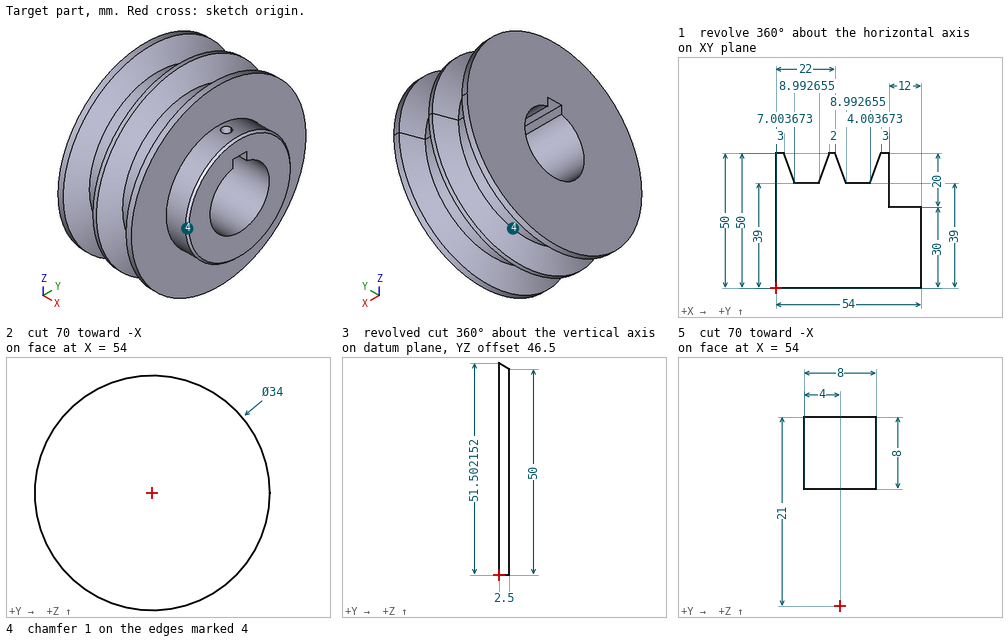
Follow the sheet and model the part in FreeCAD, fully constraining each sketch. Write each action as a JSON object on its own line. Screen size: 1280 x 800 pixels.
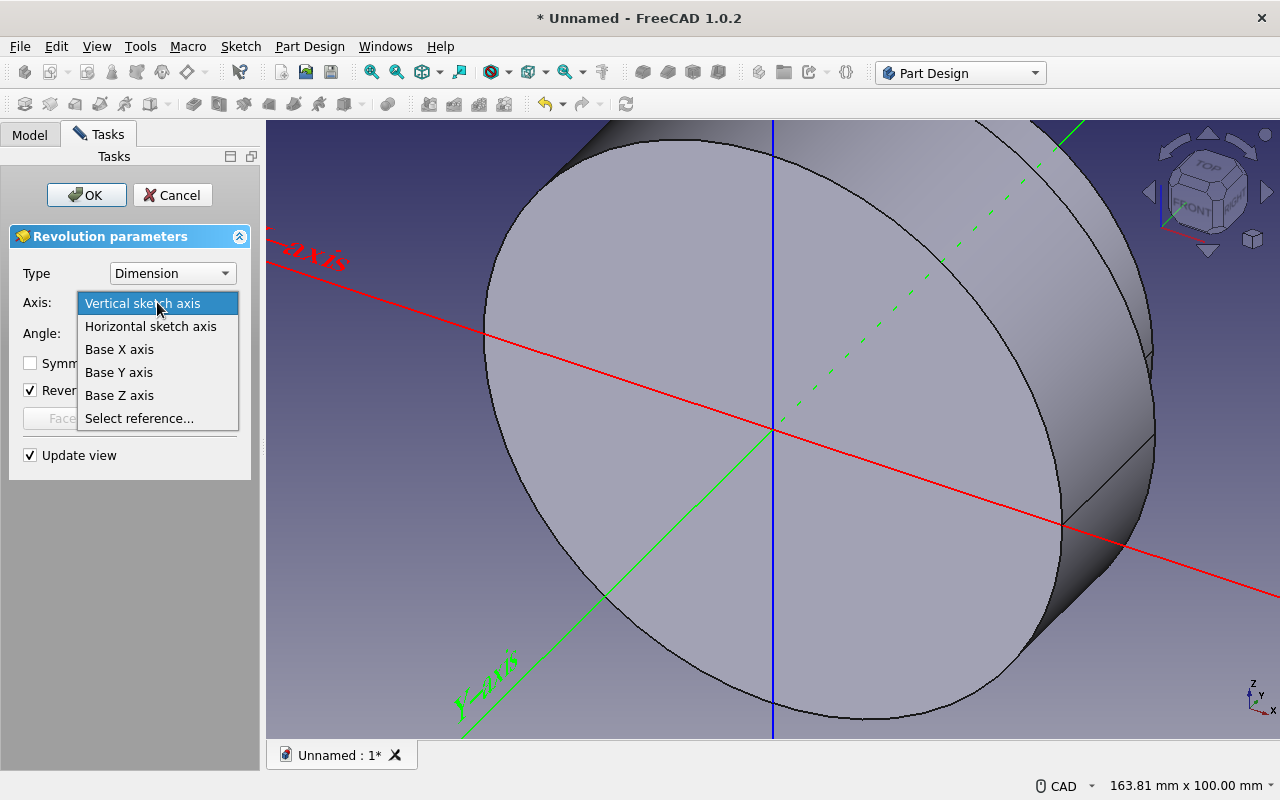
{"action": "left_click", "coordinate": [156, 326]}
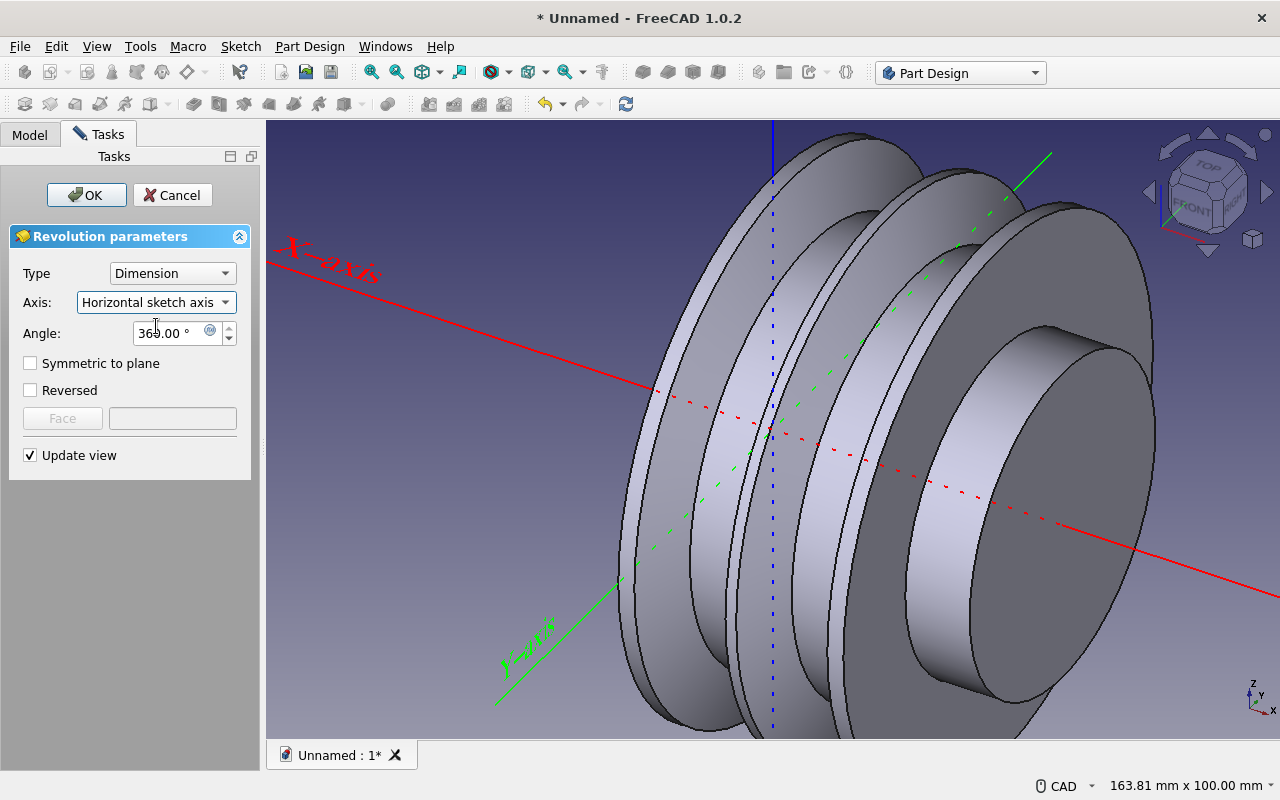
{"action": "left_click", "coordinate": [87, 195]}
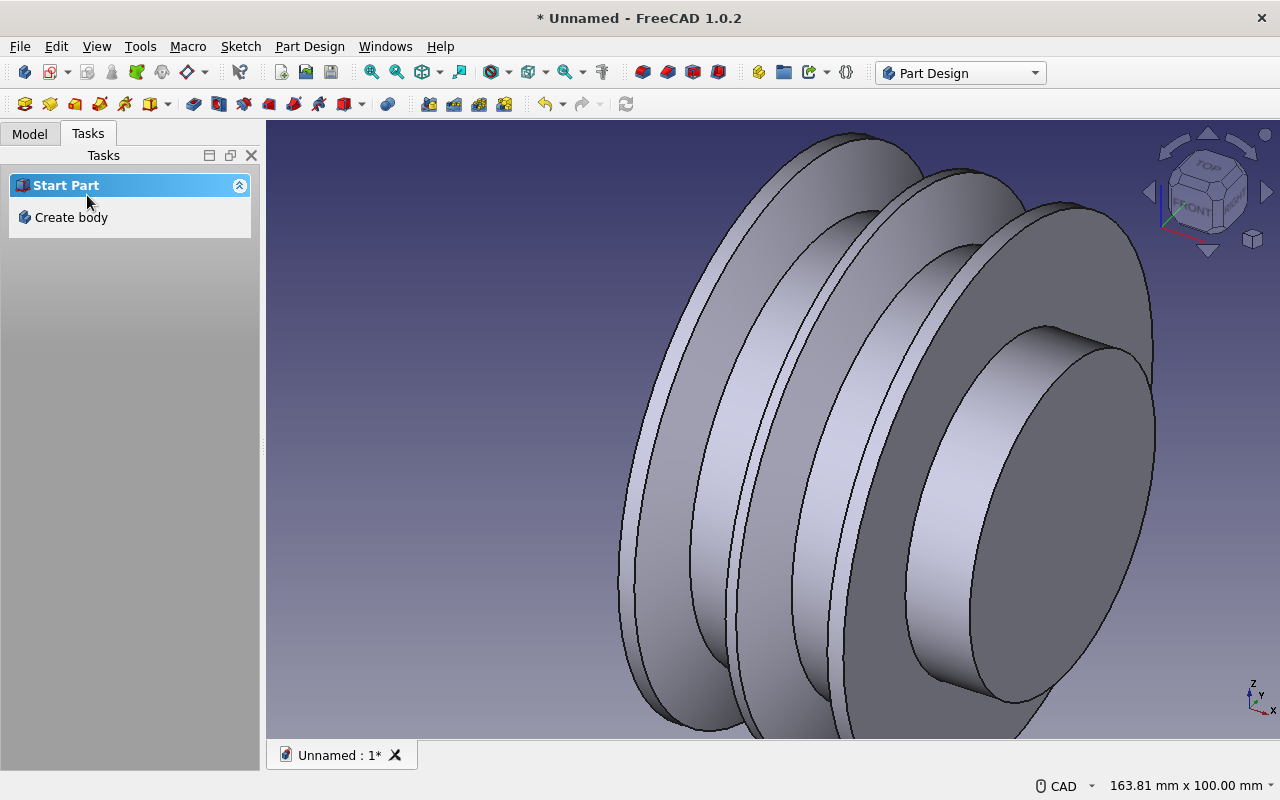
{"action": "key", "text": "v f"}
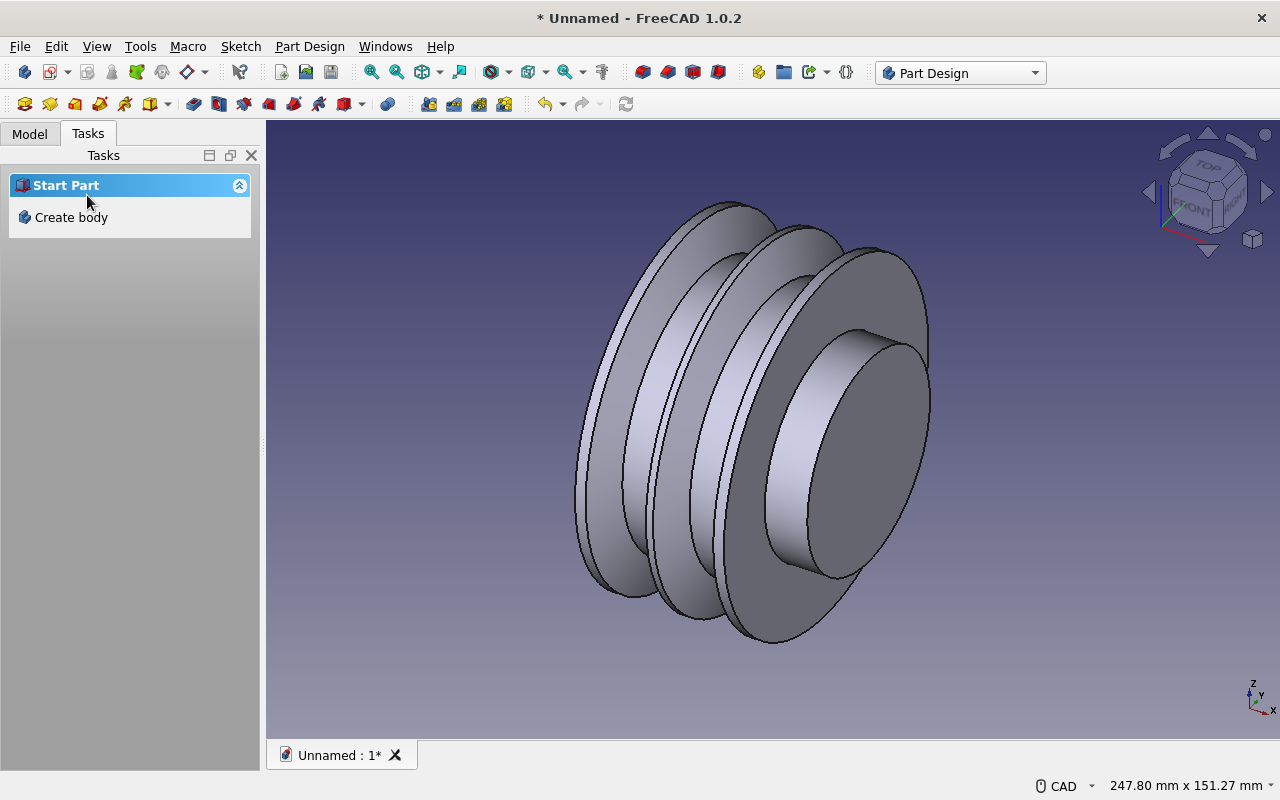
{"action": "left_click", "coordinate": [869, 460]}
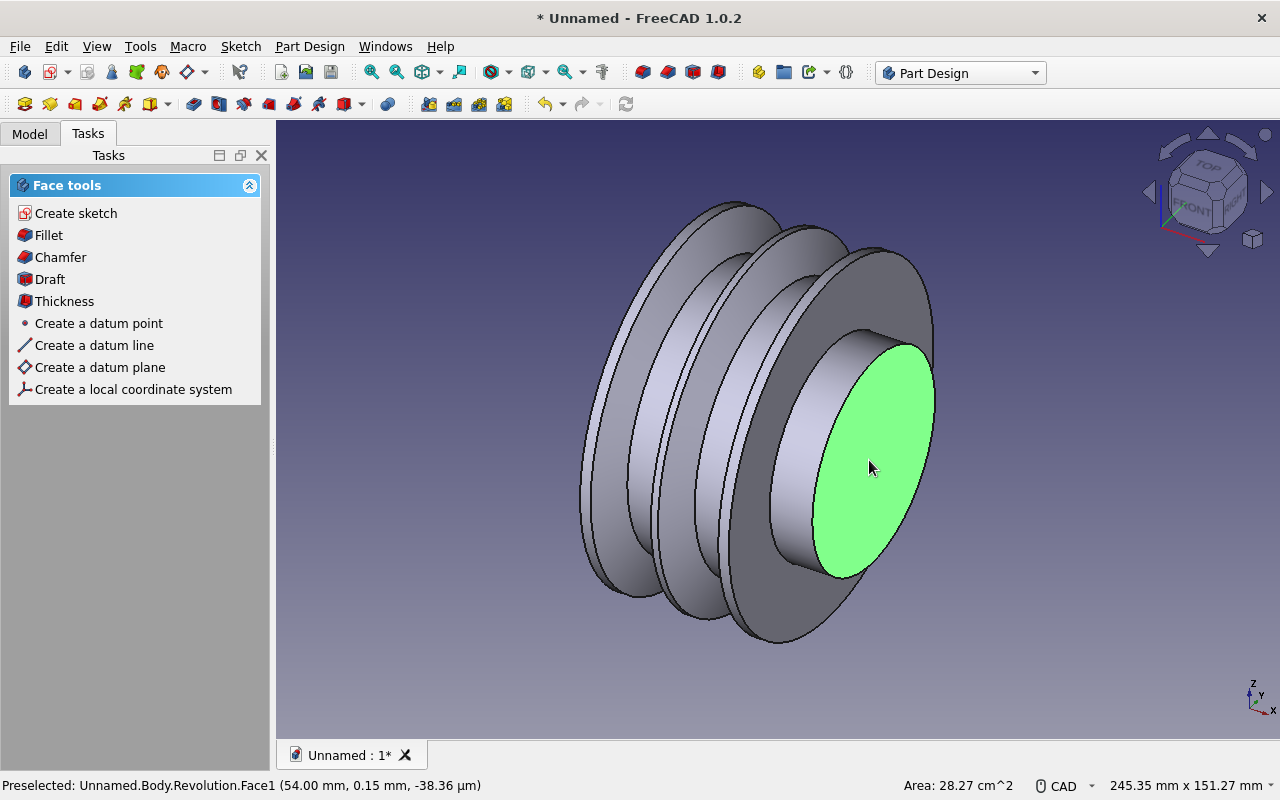
{"action": "left_click", "coordinate": [50, 72]}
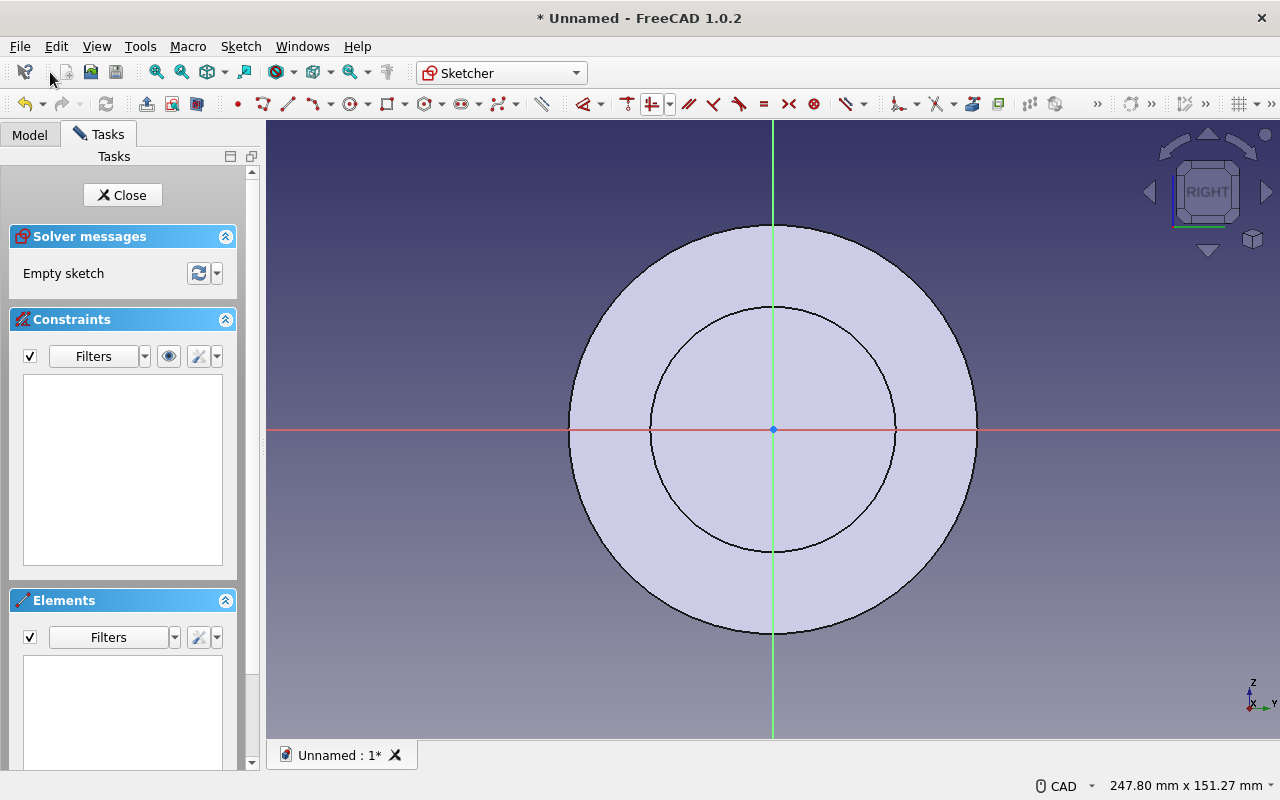
{"action": "scroll", "coordinate": [813, 429], "scroll_direction": "up", "scroll_amount": 5}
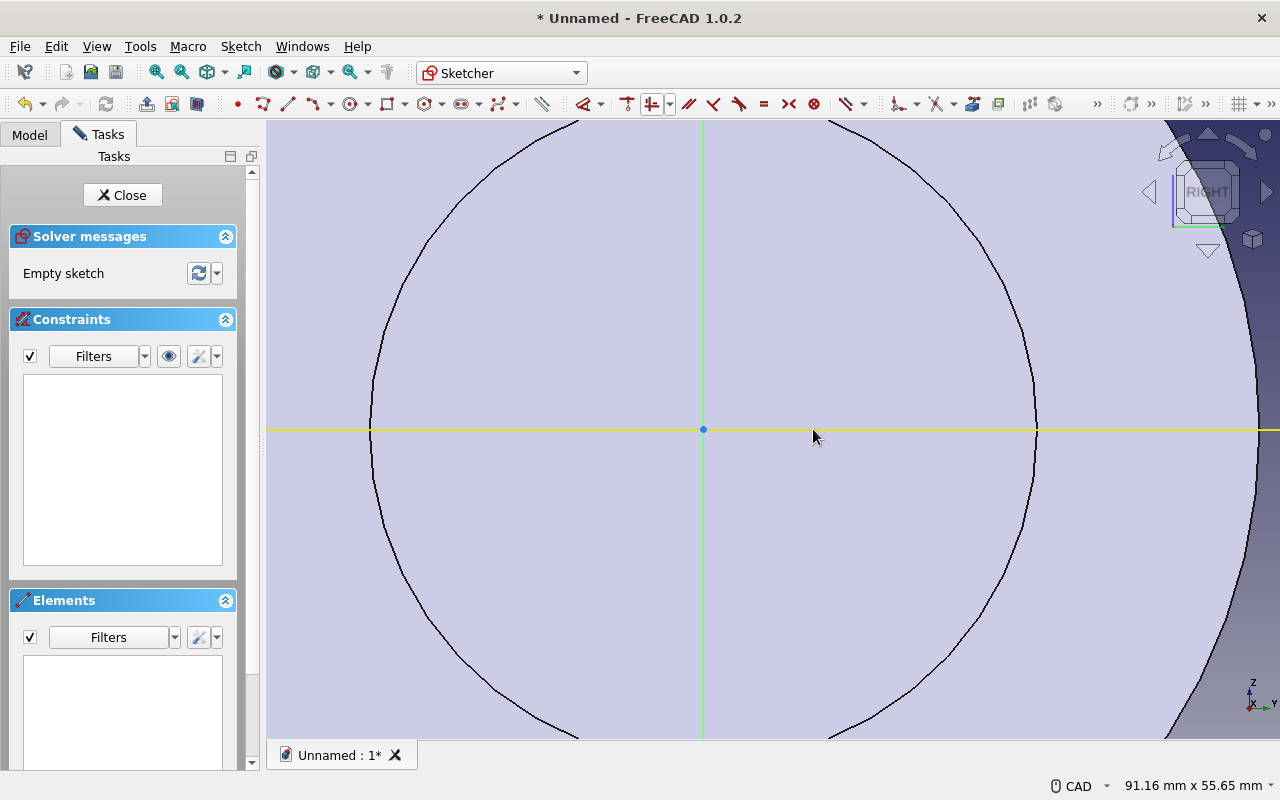
{"action": "key", "text": "g c"}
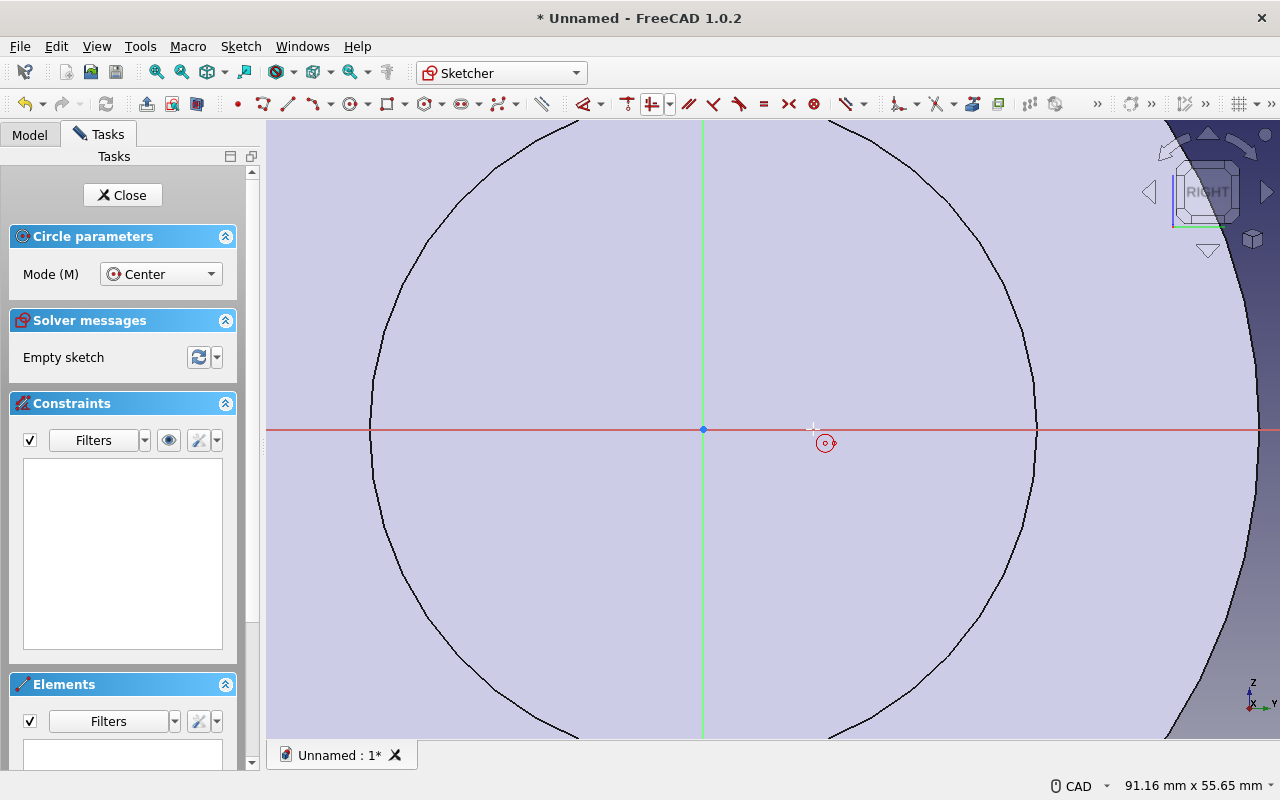
{"action": "left_click", "coordinate": [703, 430]}
{"action": "mouse_move", "coordinate": [837, 296]}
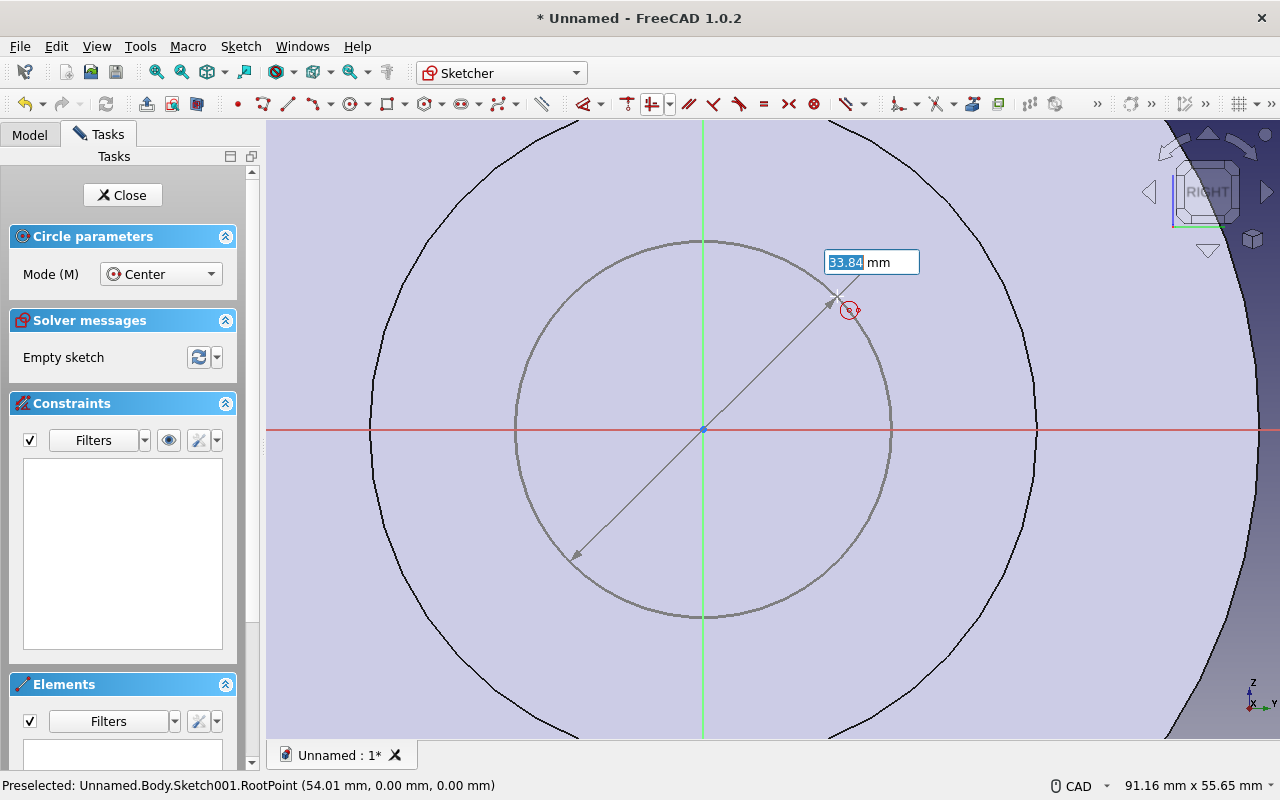
{"action": "type", "text": "34"}
{"action": "key", "text": "Return"}
{"action": "key", "text": "Escape"}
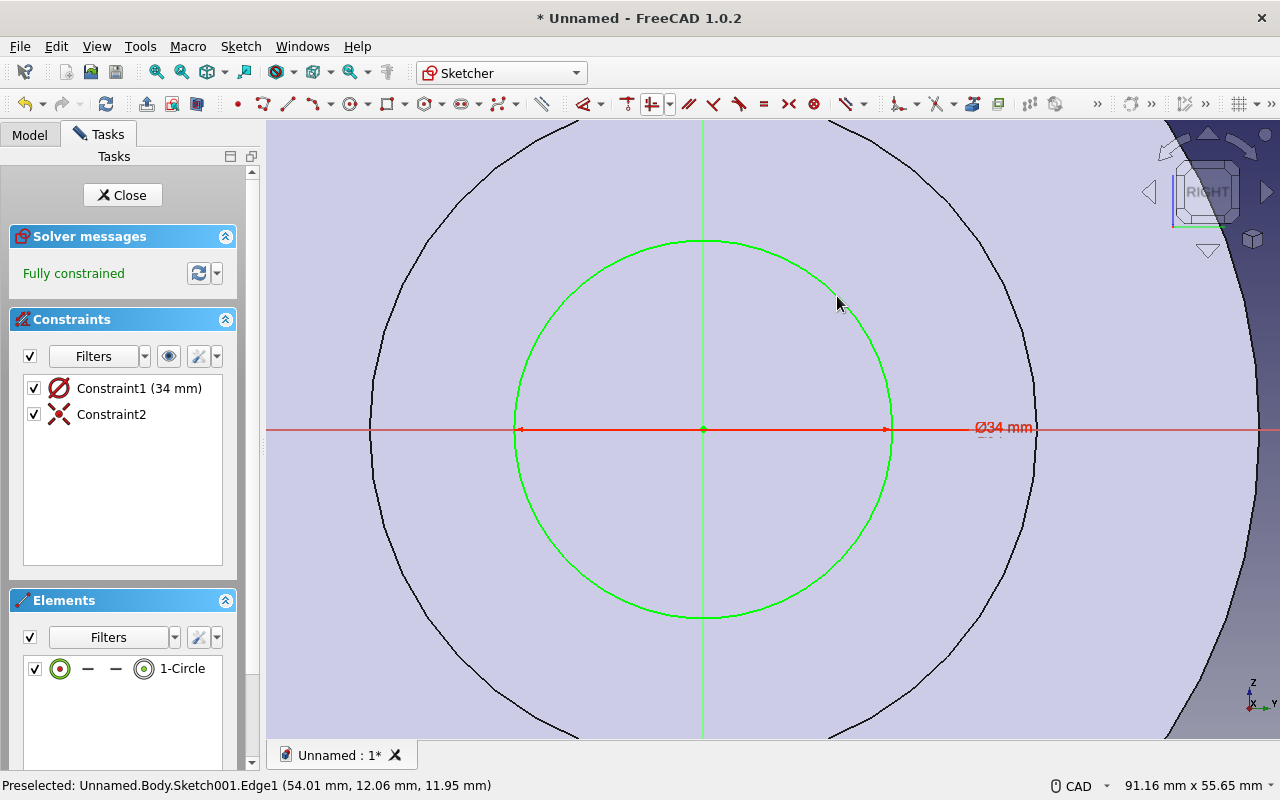
{"action": "left_click", "coordinate": [123, 195]}